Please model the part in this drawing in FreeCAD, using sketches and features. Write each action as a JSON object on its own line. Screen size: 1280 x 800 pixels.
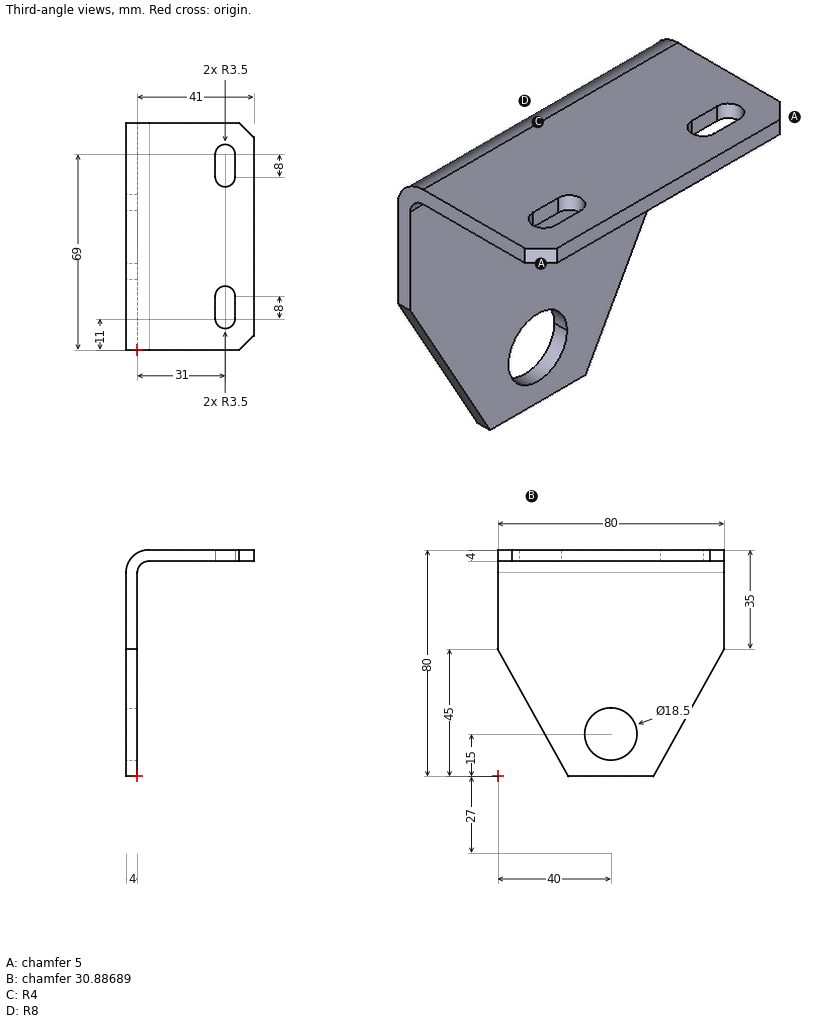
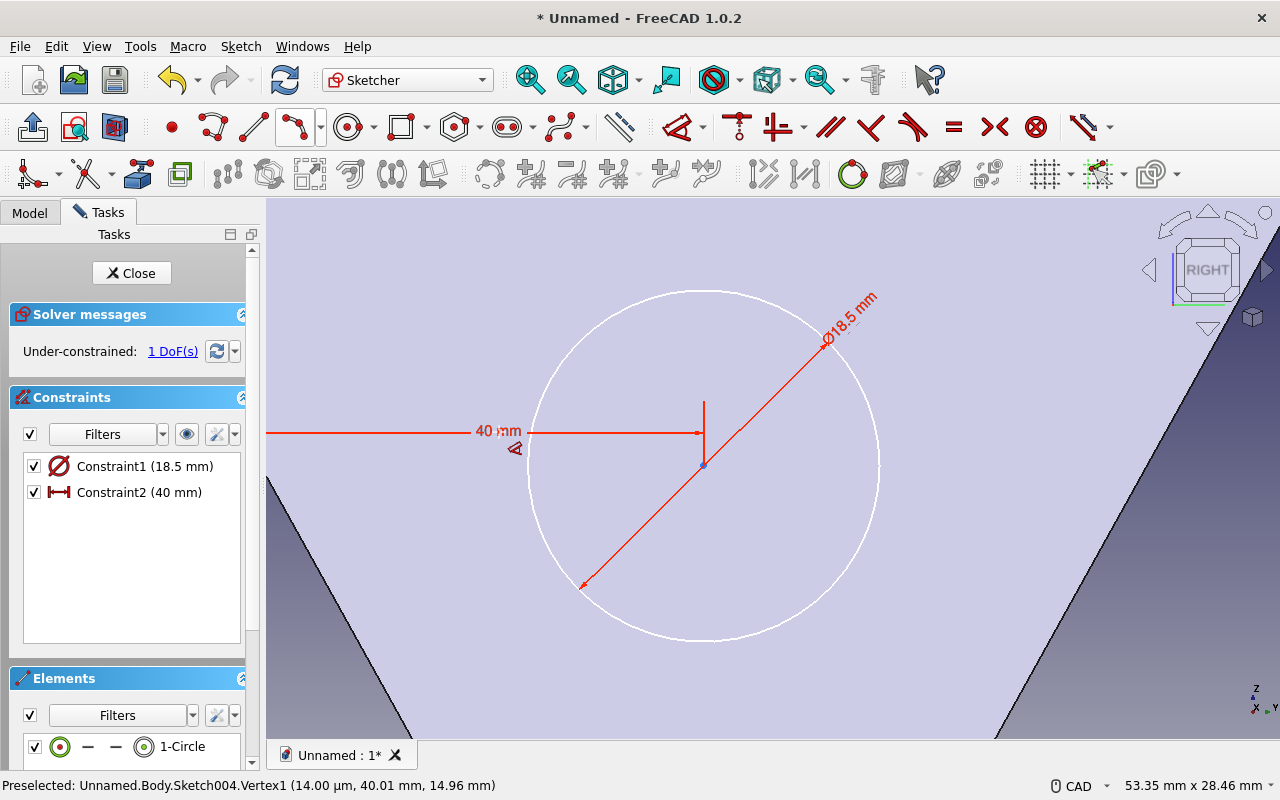
{"action": "left_click", "coordinate": [704, 466]}
{"action": "left_click", "coordinate": [738, 589]}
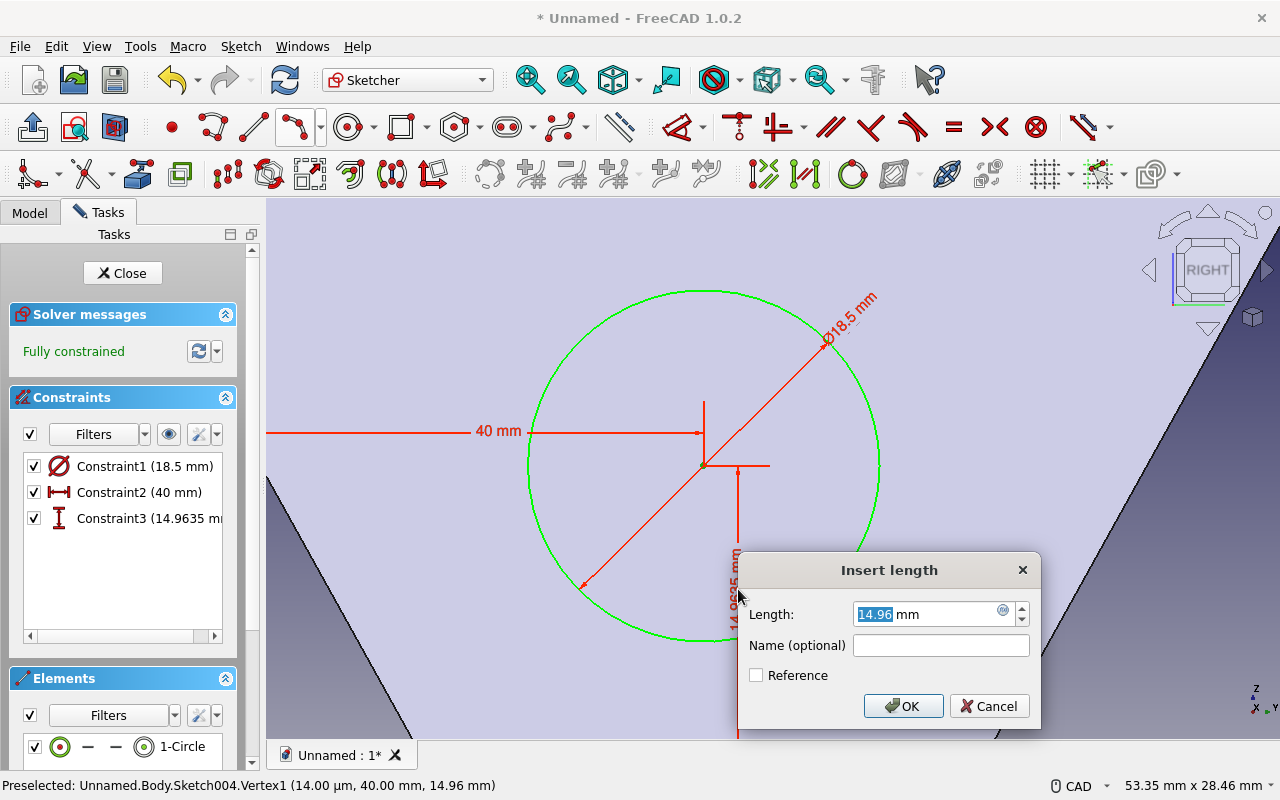
{"action": "type", "text": "15"}
{"action": "key", "text": "Return"}
{"action": "key", "text": "Escape"}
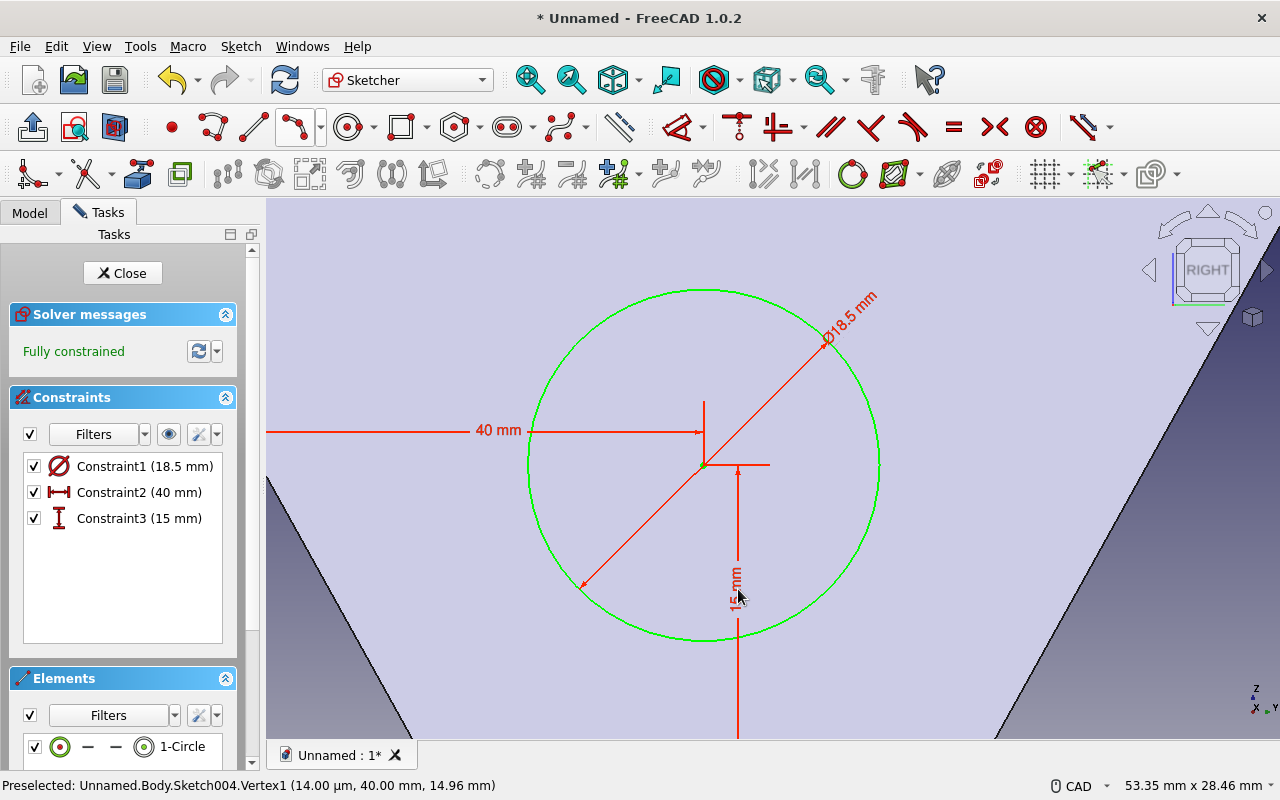
{"action": "left_click", "coordinate": [123, 273]}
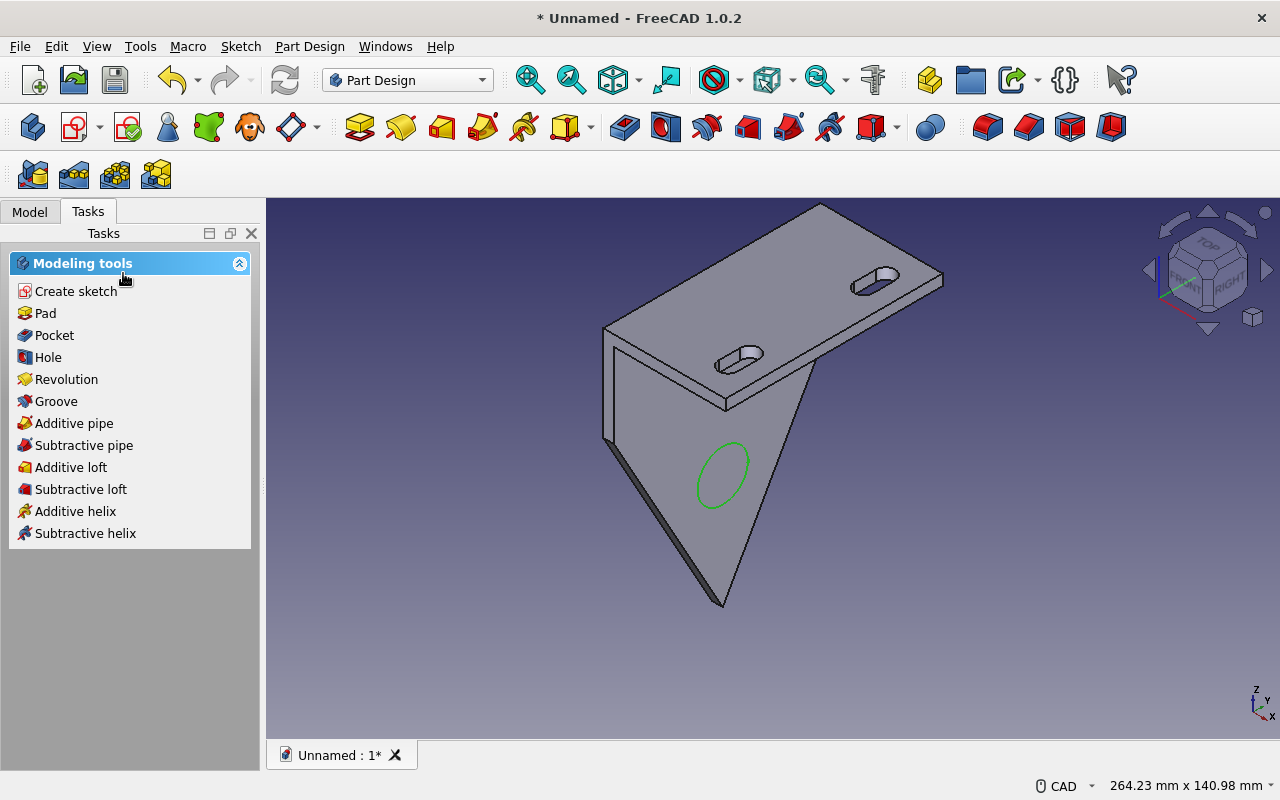
{"action": "left_click", "coordinate": [625, 128]}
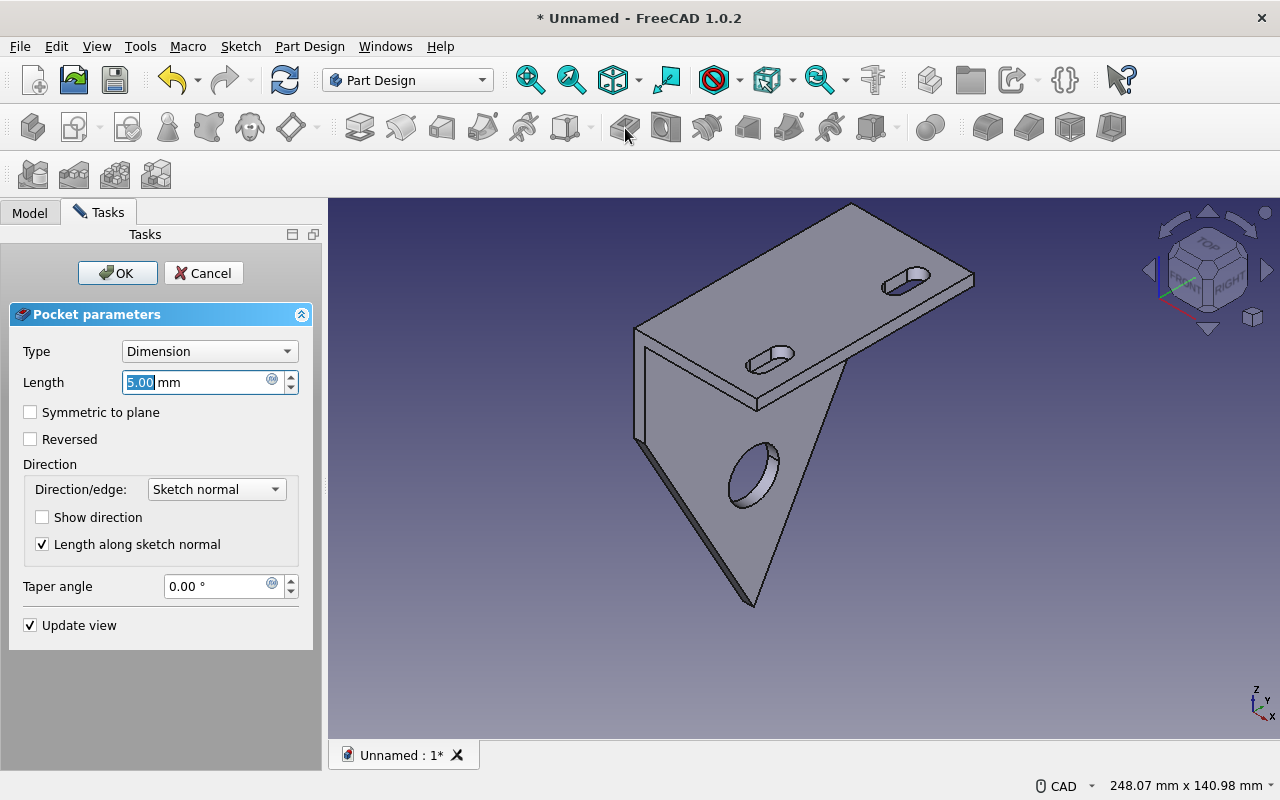
{"action": "left_click", "coordinate": [210, 352]}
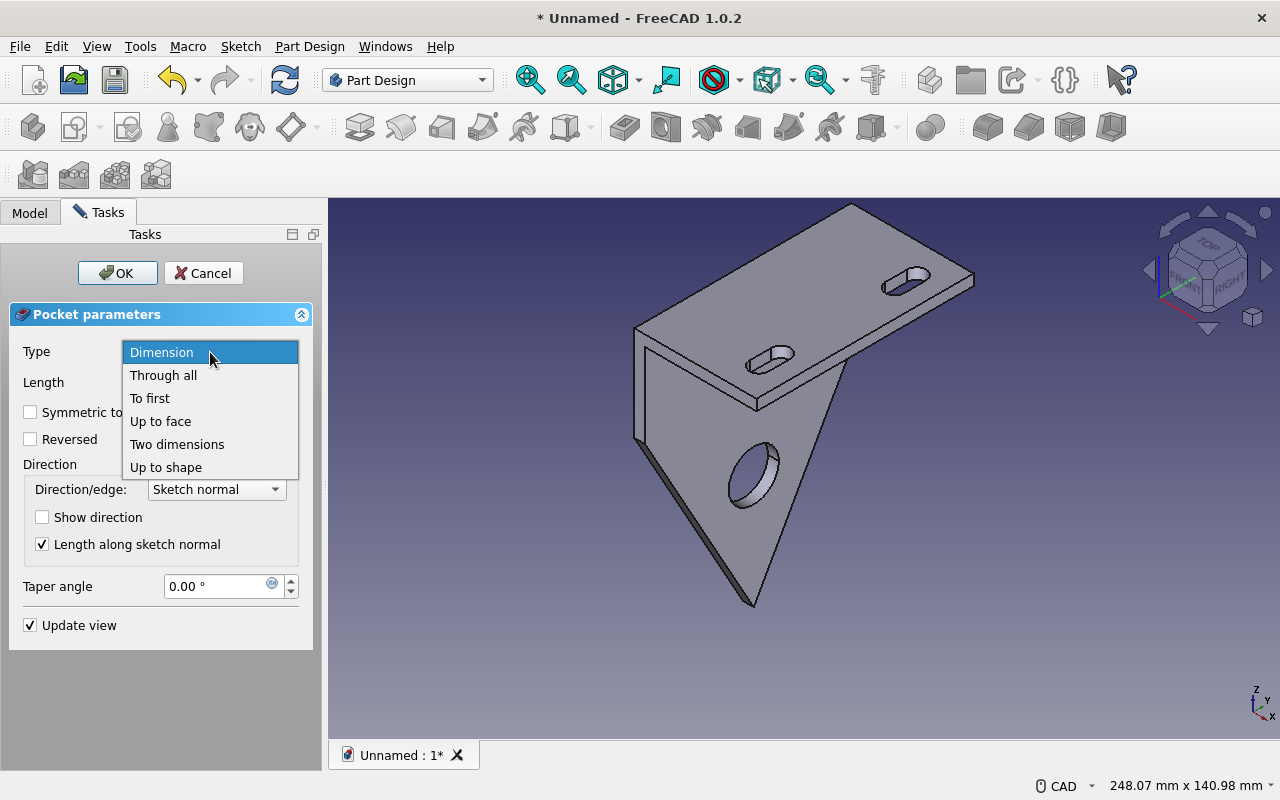
{"action": "left_click", "coordinate": [208, 376]}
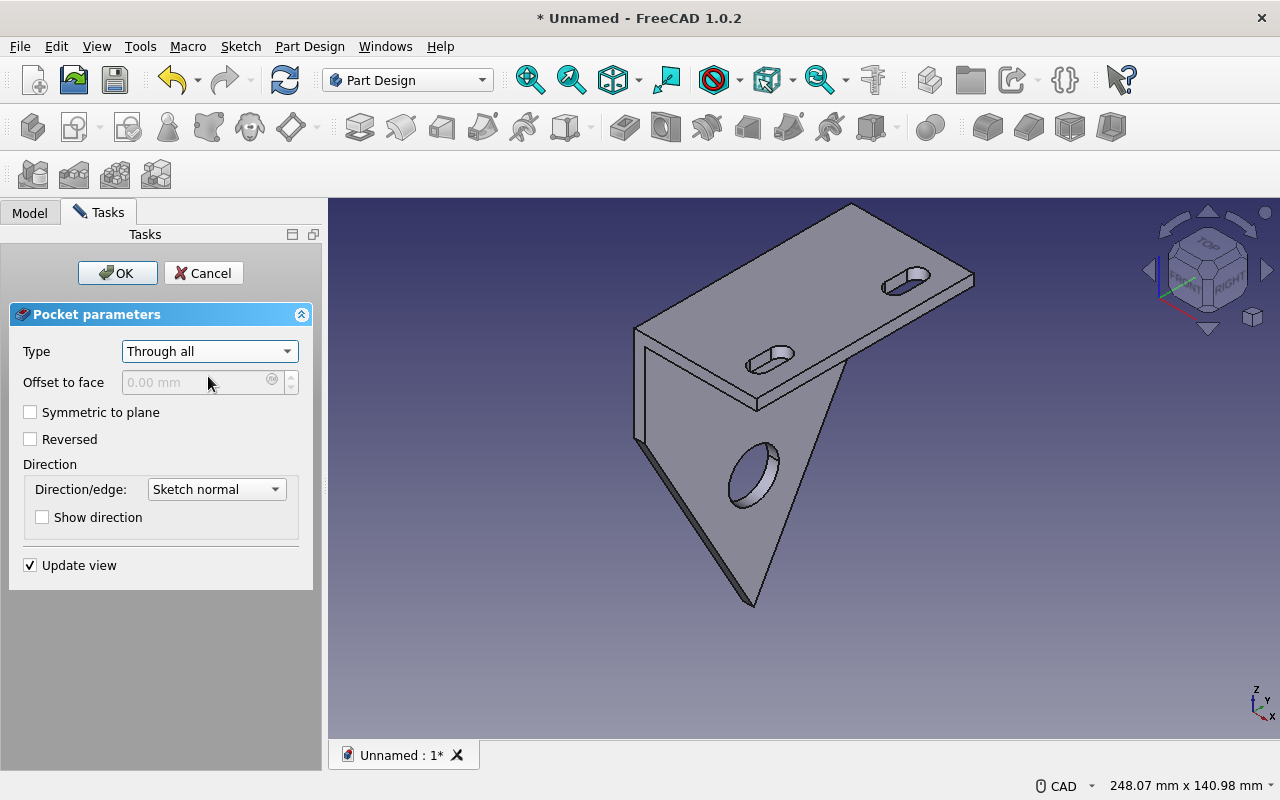
{"action": "left_click", "coordinate": [118, 273]}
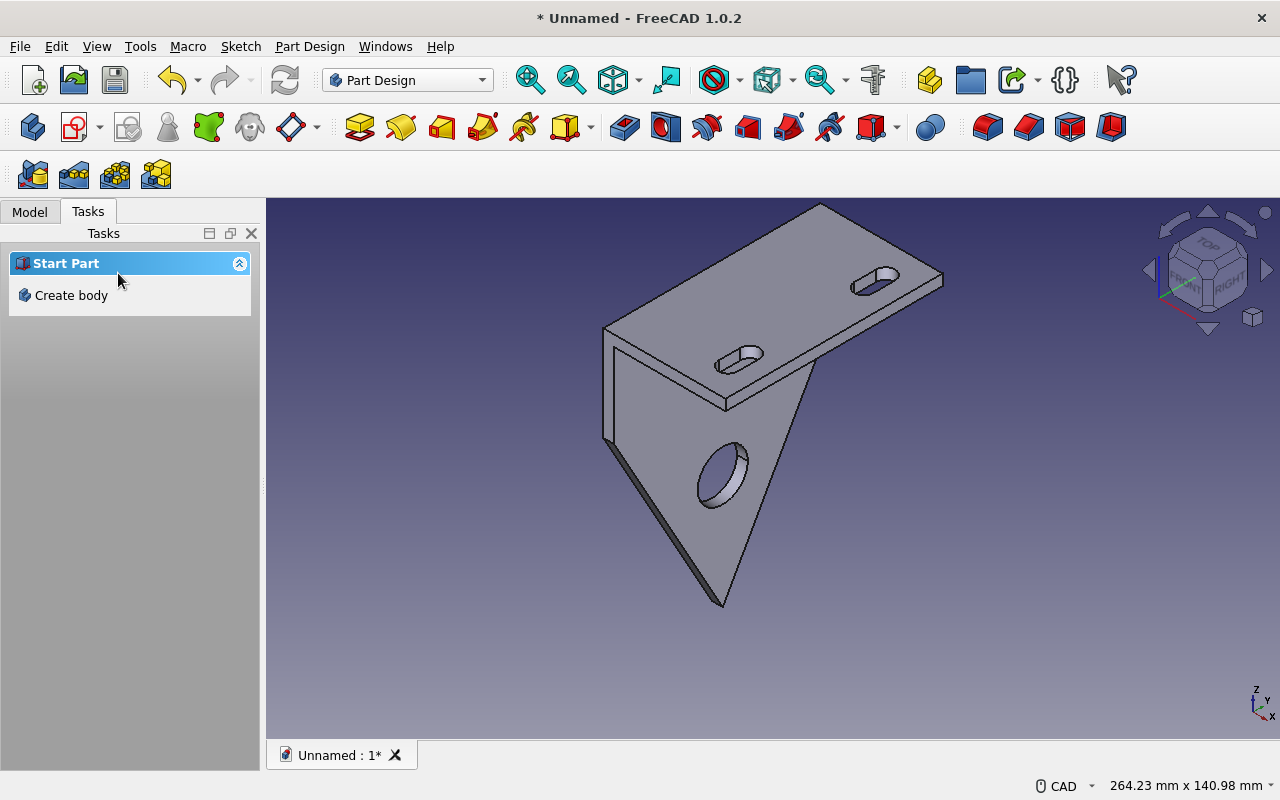
{"action": "left_click", "coordinate": [726, 404]}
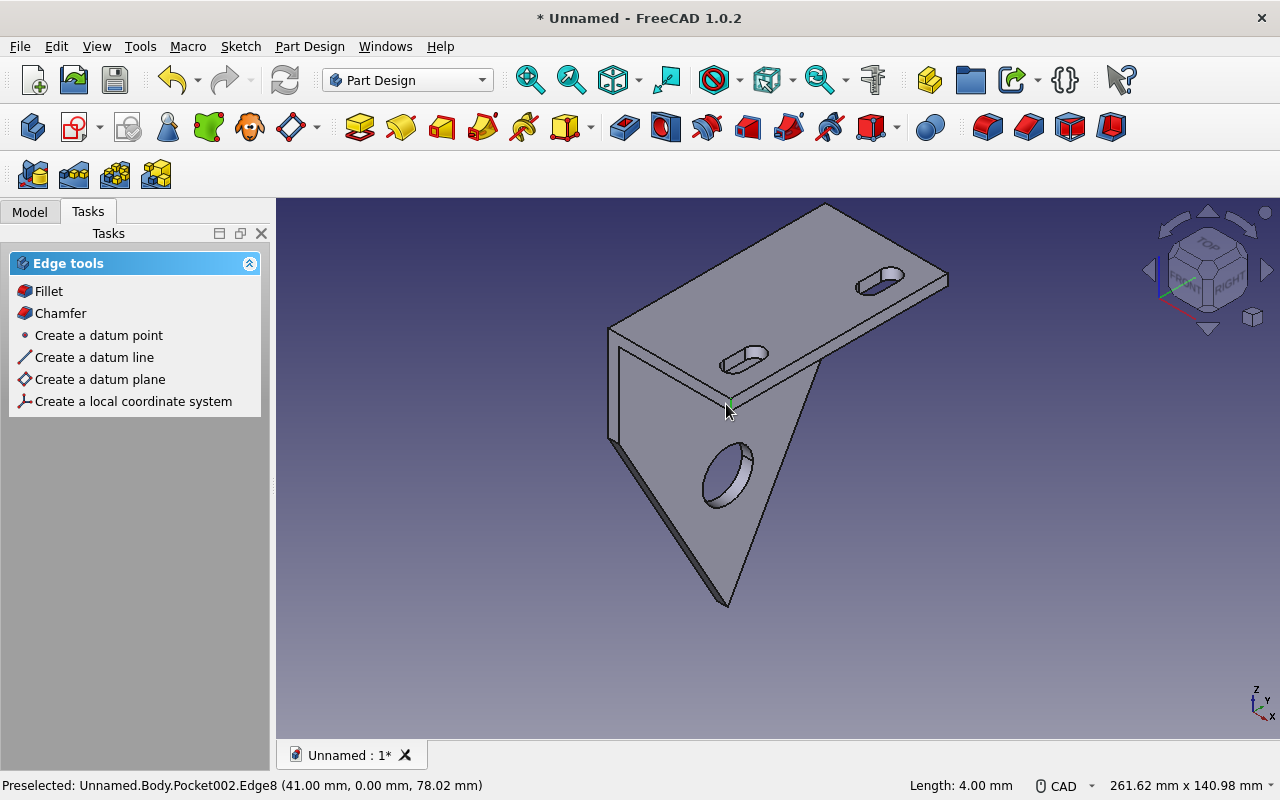
{"action": "scroll", "coordinate": [948, 279], "scroll_direction": "up", "scroll_amount": 5}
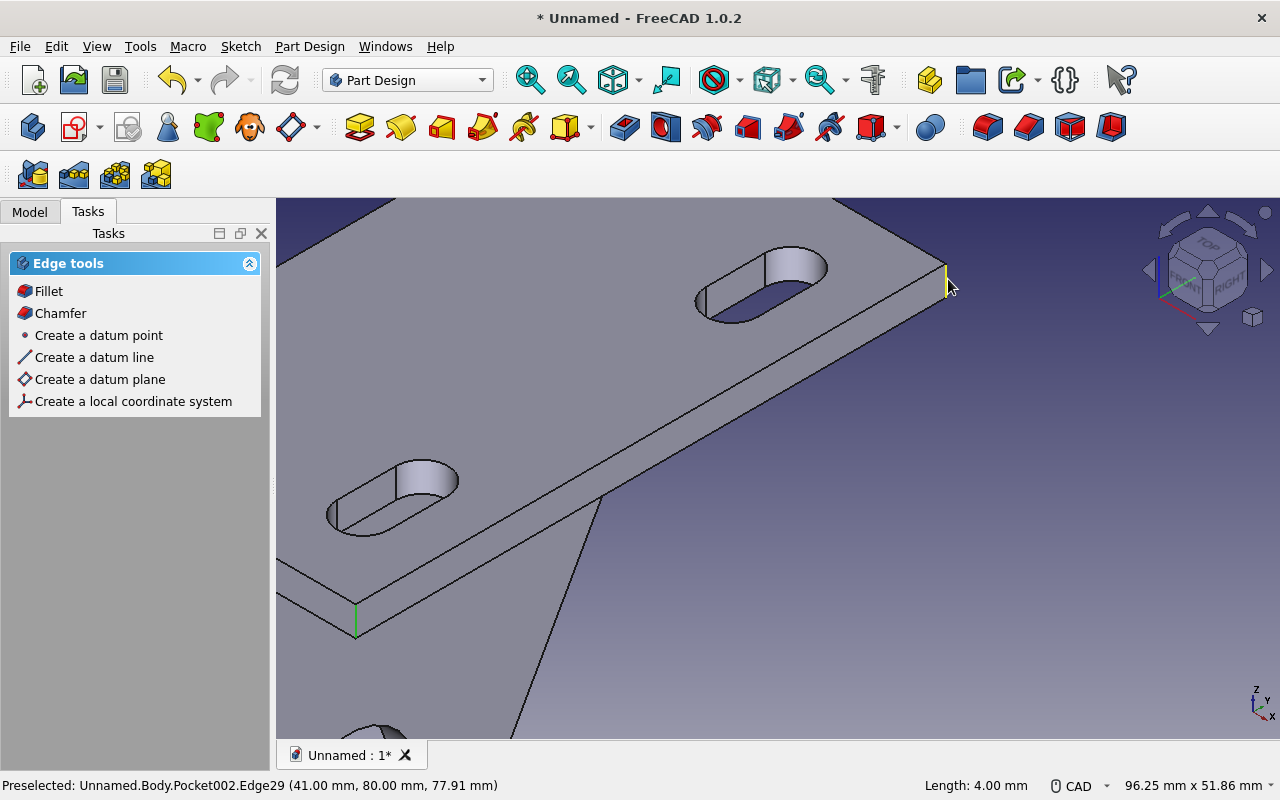
{"action": "key", "text": "v f"}